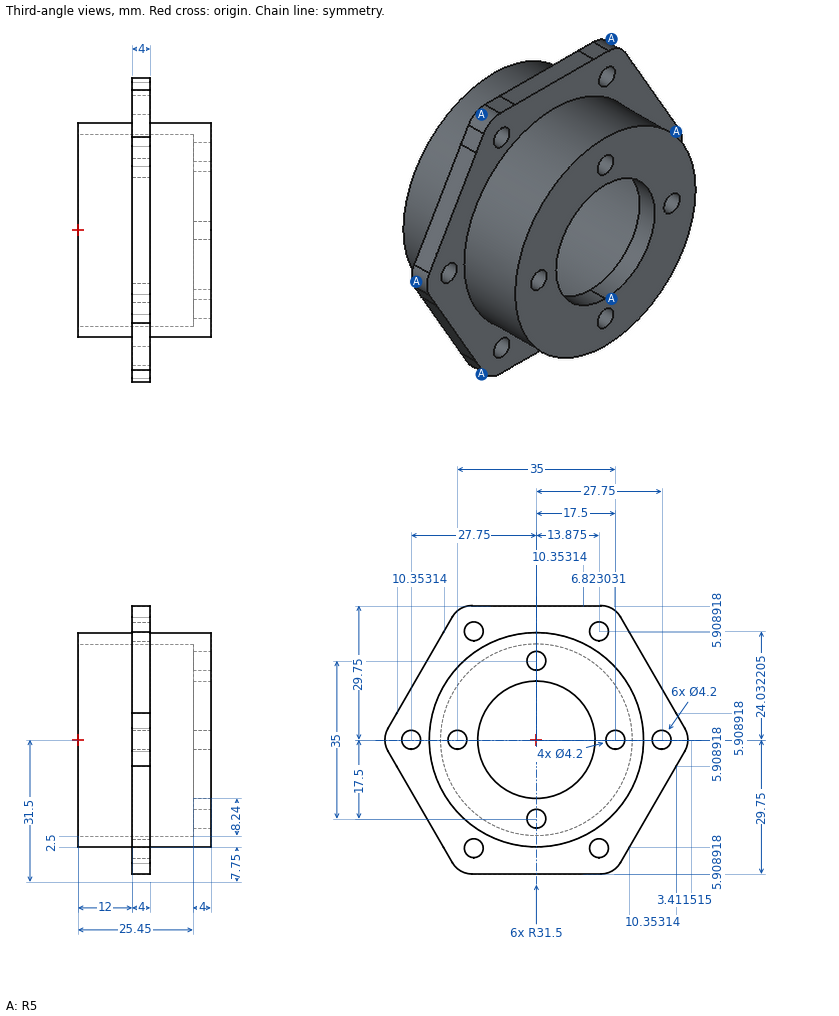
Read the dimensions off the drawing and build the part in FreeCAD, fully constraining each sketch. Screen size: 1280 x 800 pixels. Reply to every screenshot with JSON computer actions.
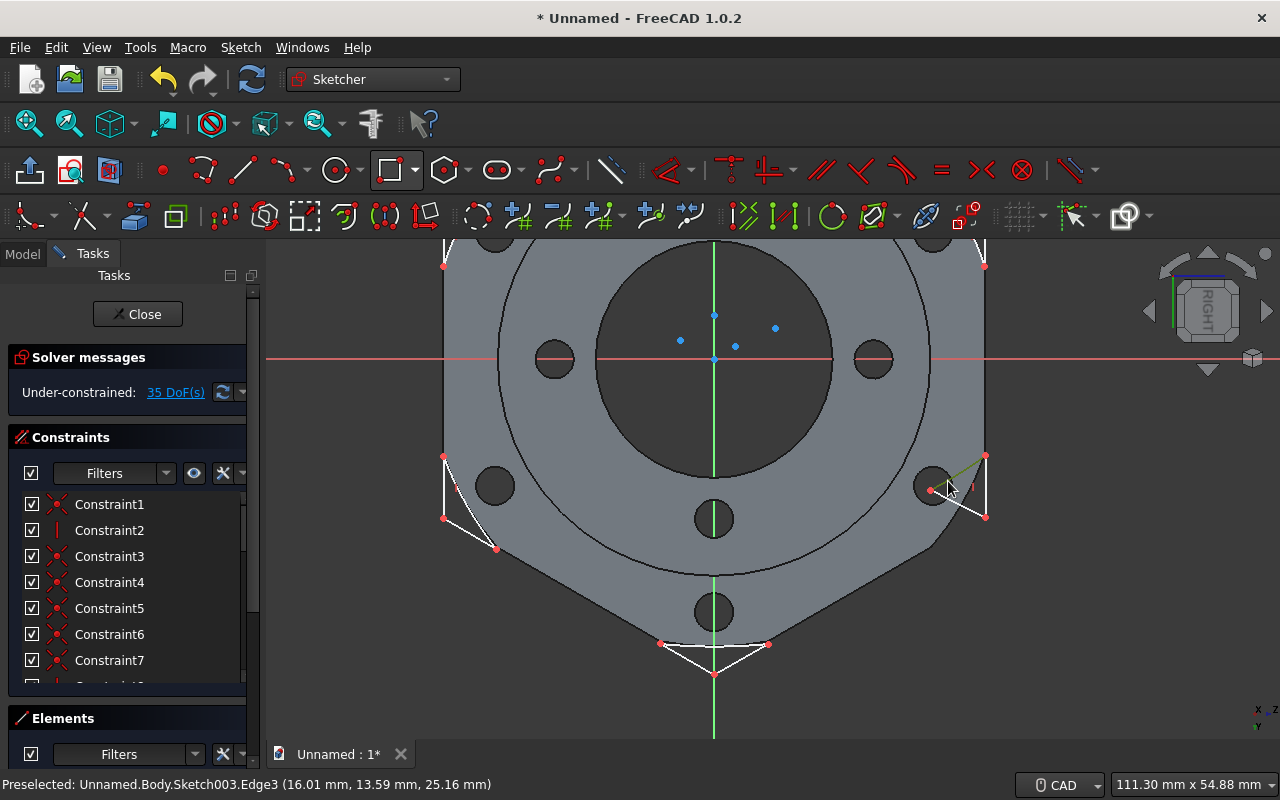
{"action": "left_click", "coordinate": [478, 523]}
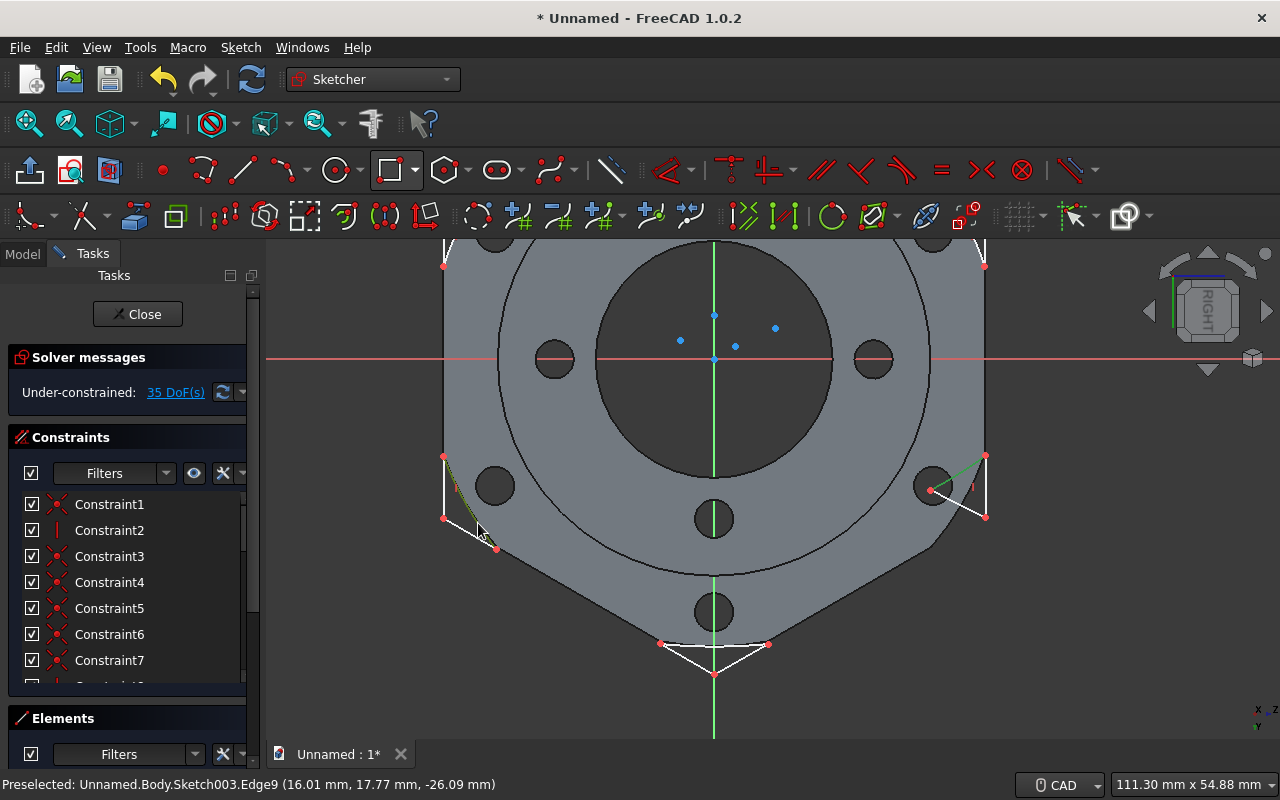
{"action": "left_click", "coordinate": [730, 170]}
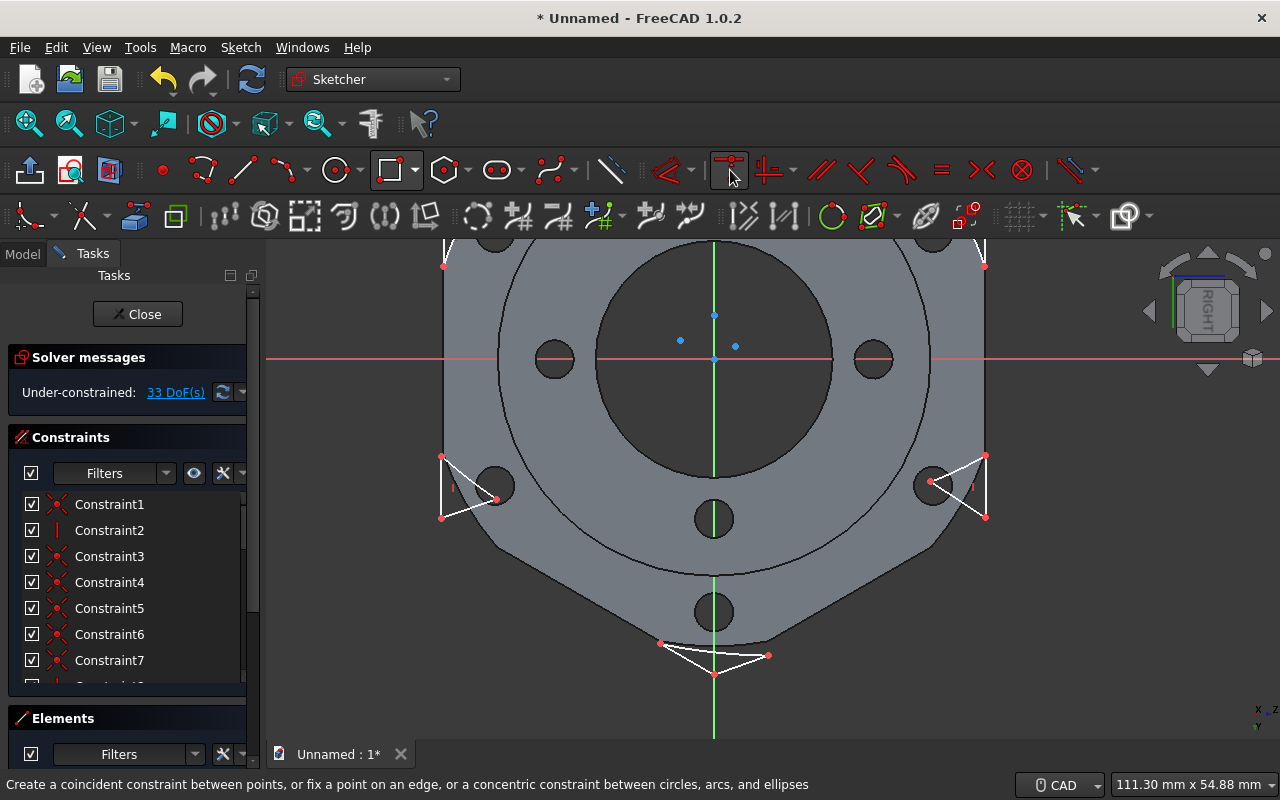
{"action": "left_click", "coordinate": [948, 475]}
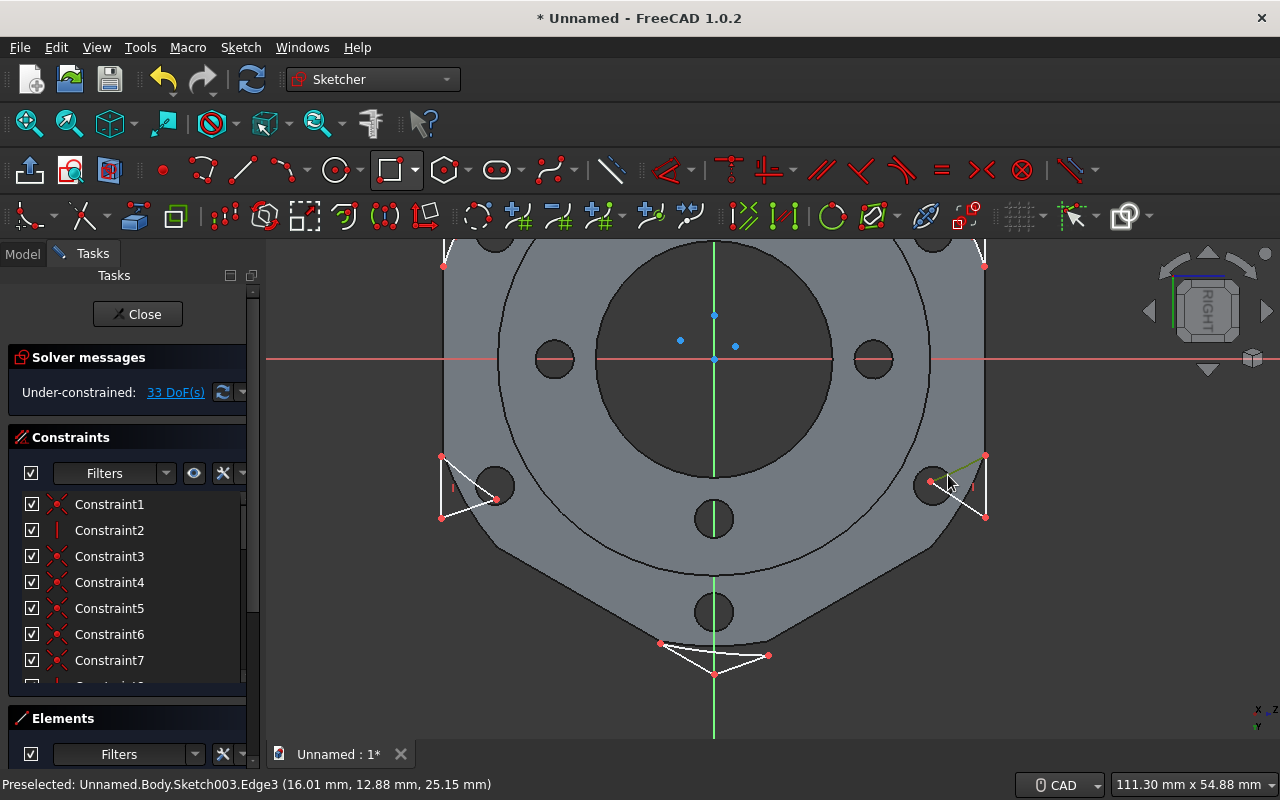
{"action": "scroll", "coordinate": [693, 647], "scroll_direction": "down", "scroll_amount": 3}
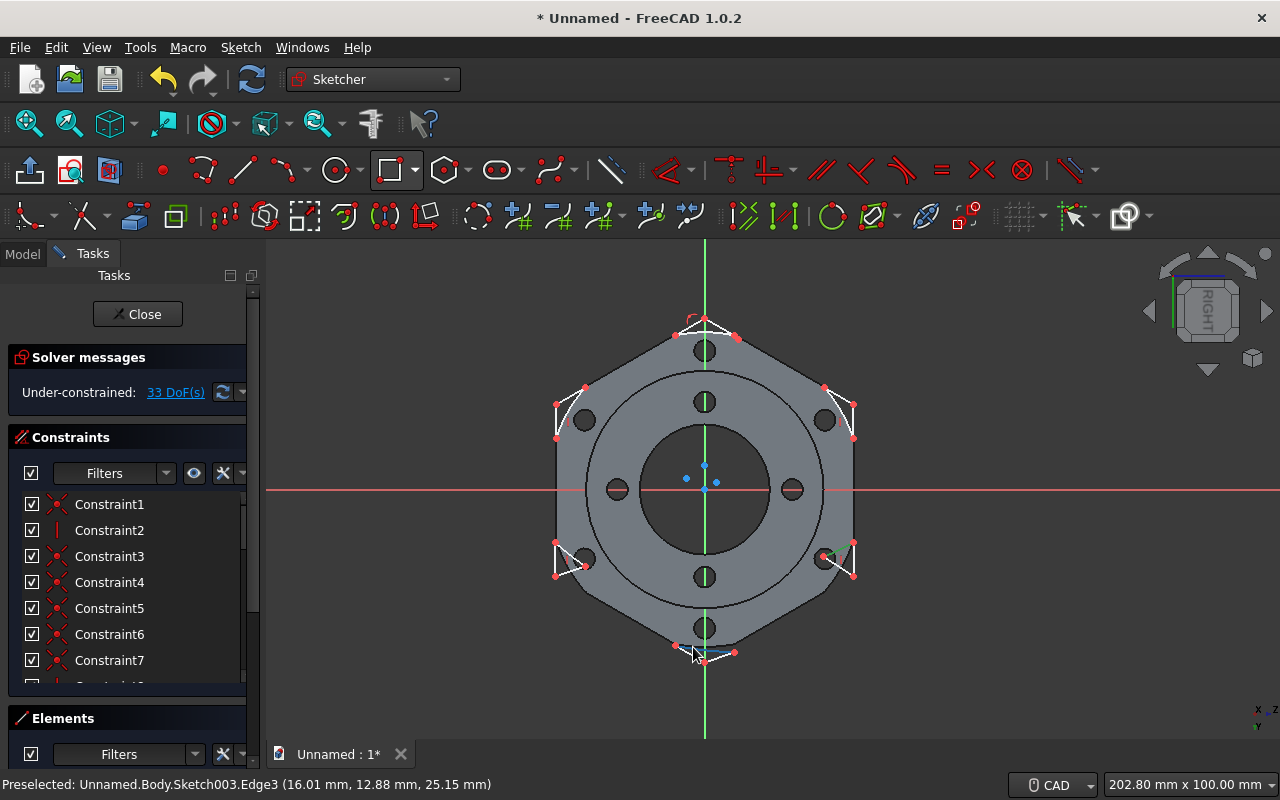
{"action": "scroll", "coordinate": [574, 402], "scroll_direction": "up", "scroll_amount": 4}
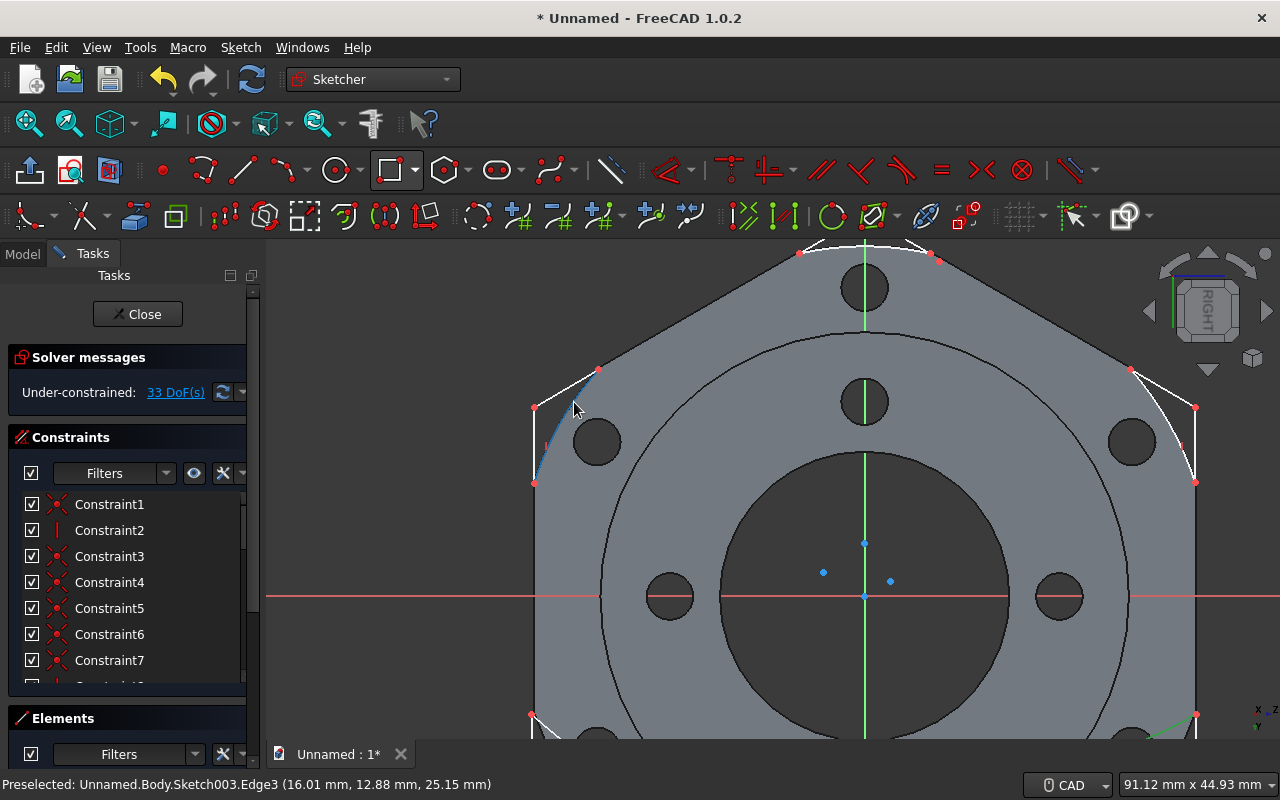
{"action": "left_click", "coordinate": [574, 401]}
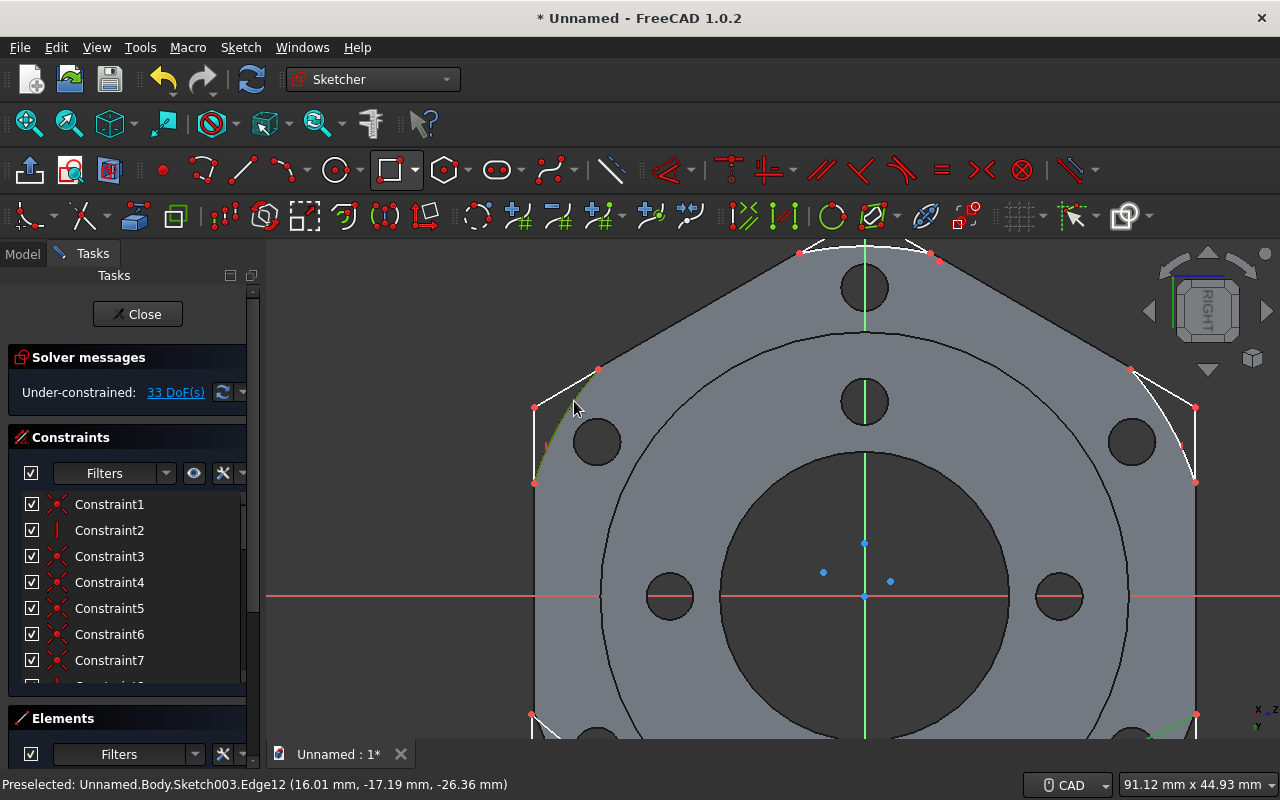
{"action": "left_click", "coordinate": [730, 170]}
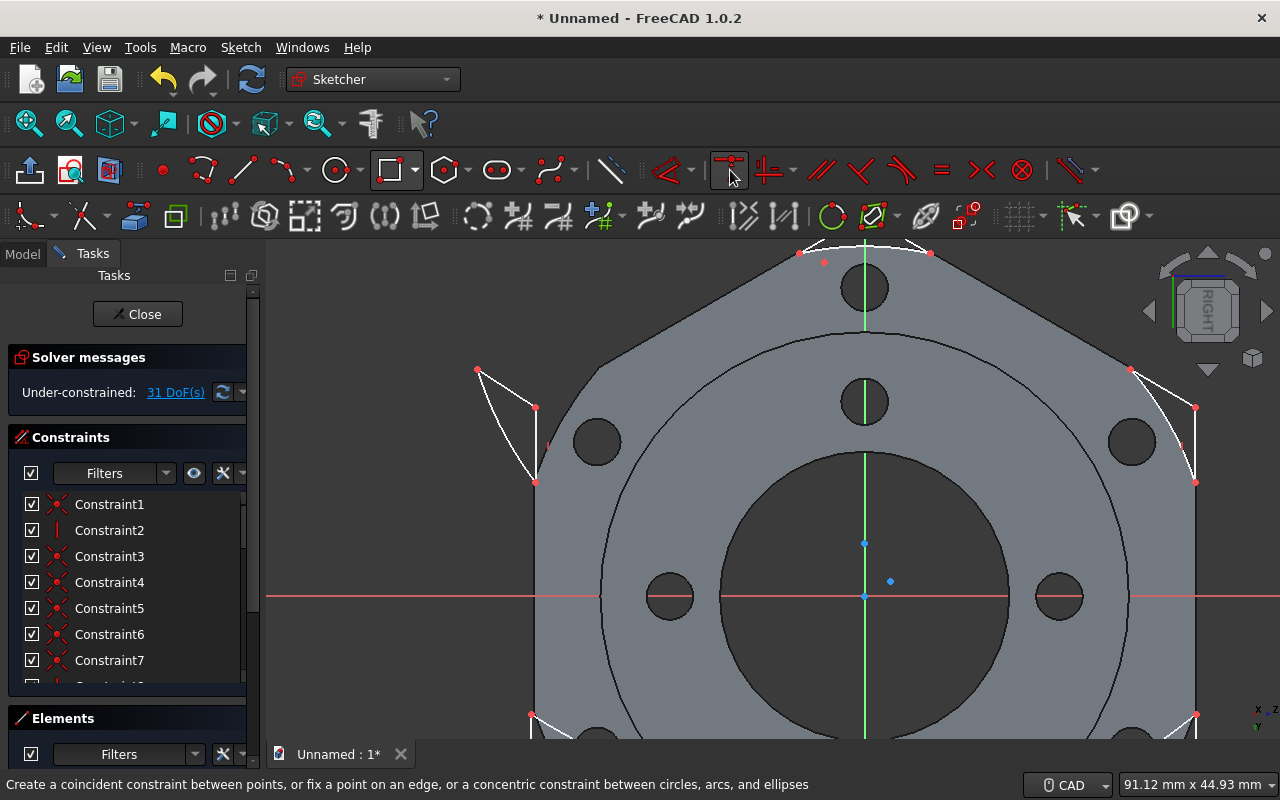
{"action": "scroll", "coordinate": [574, 401], "scroll_direction": "down", "scroll_amount": 4}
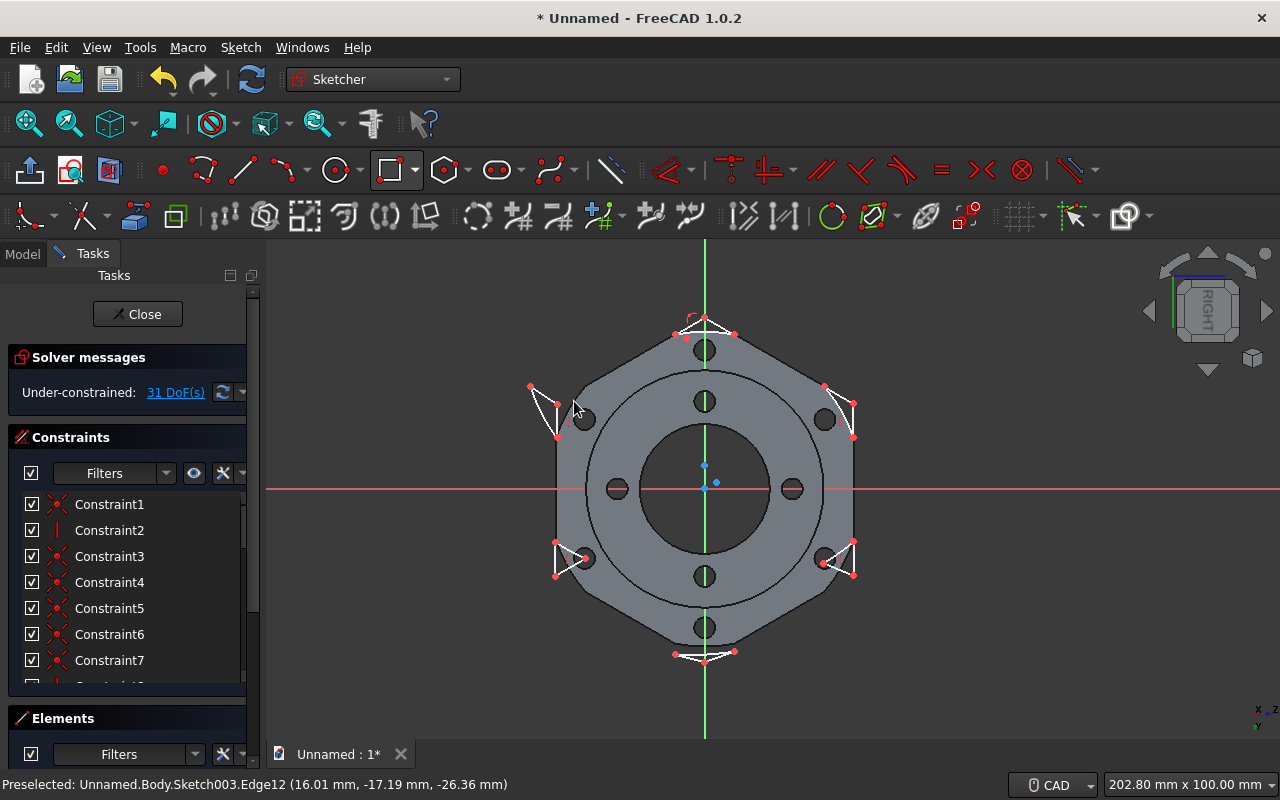
{"action": "scroll", "coordinate": [833, 557], "scroll_direction": "up", "scroll_amount": 3}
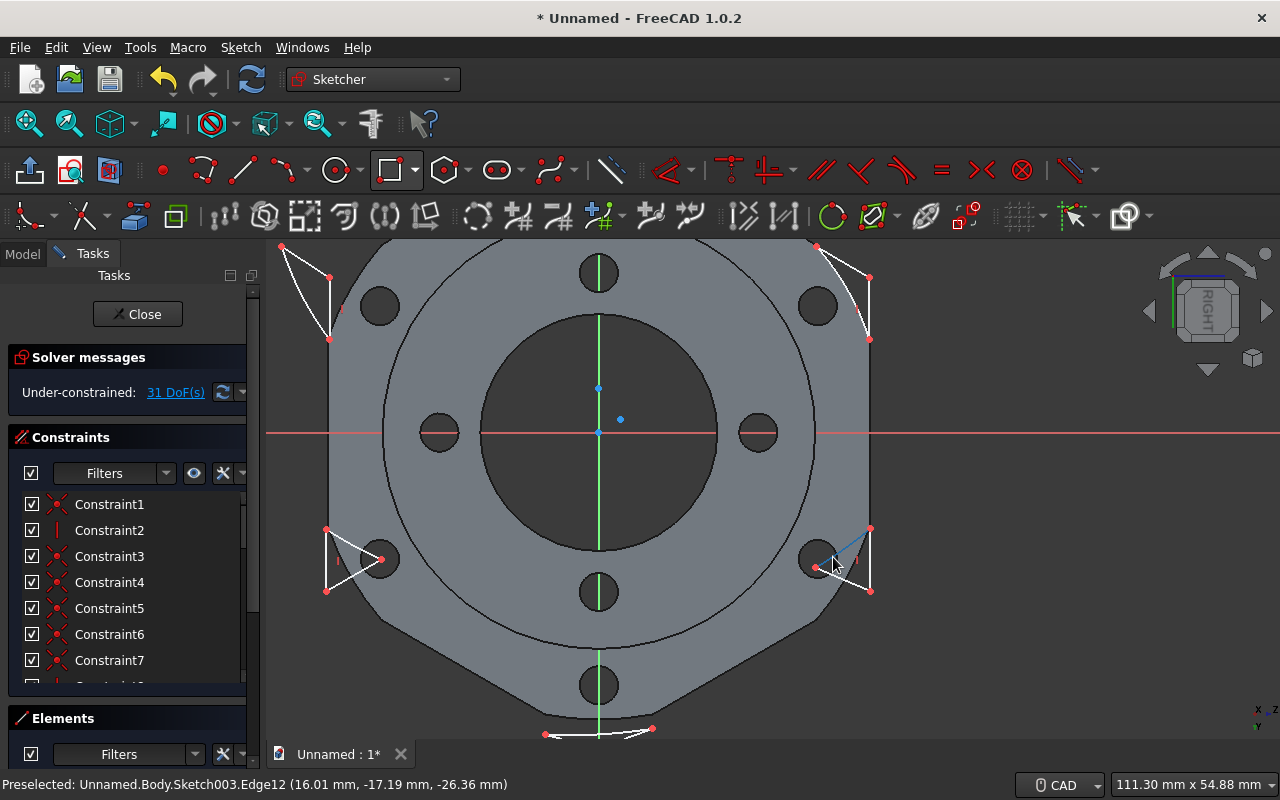
{"action": "left_click", "coordinate": [833, 557]}